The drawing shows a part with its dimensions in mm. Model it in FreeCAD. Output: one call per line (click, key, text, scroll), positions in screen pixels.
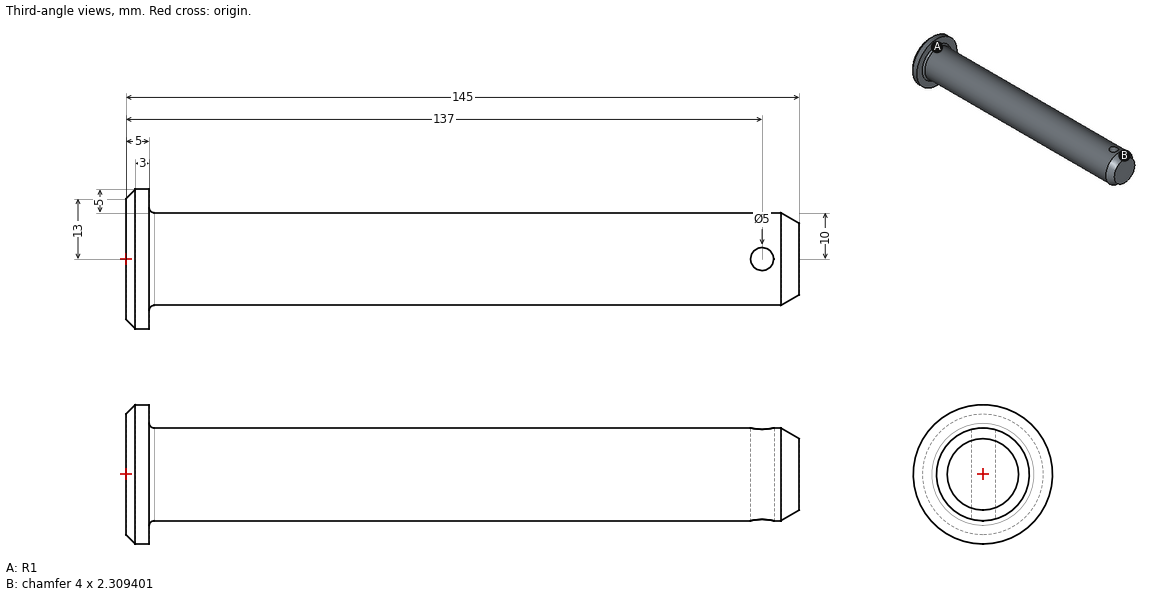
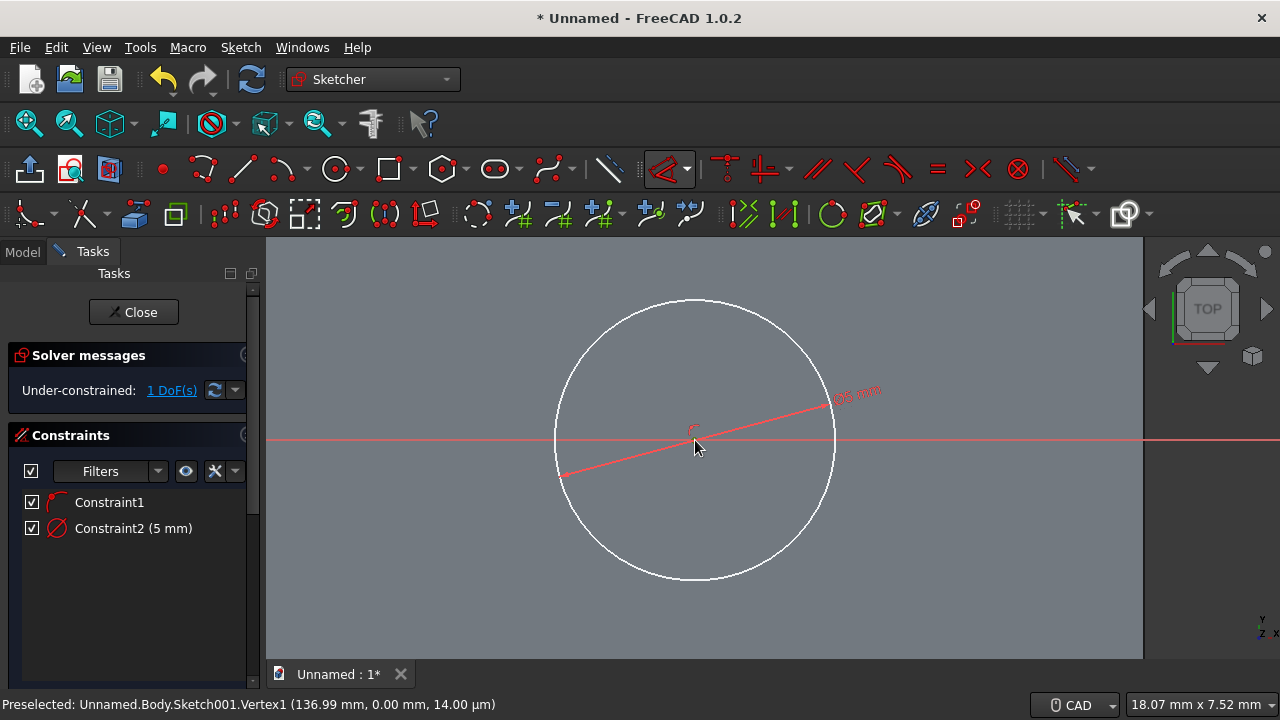
key(l)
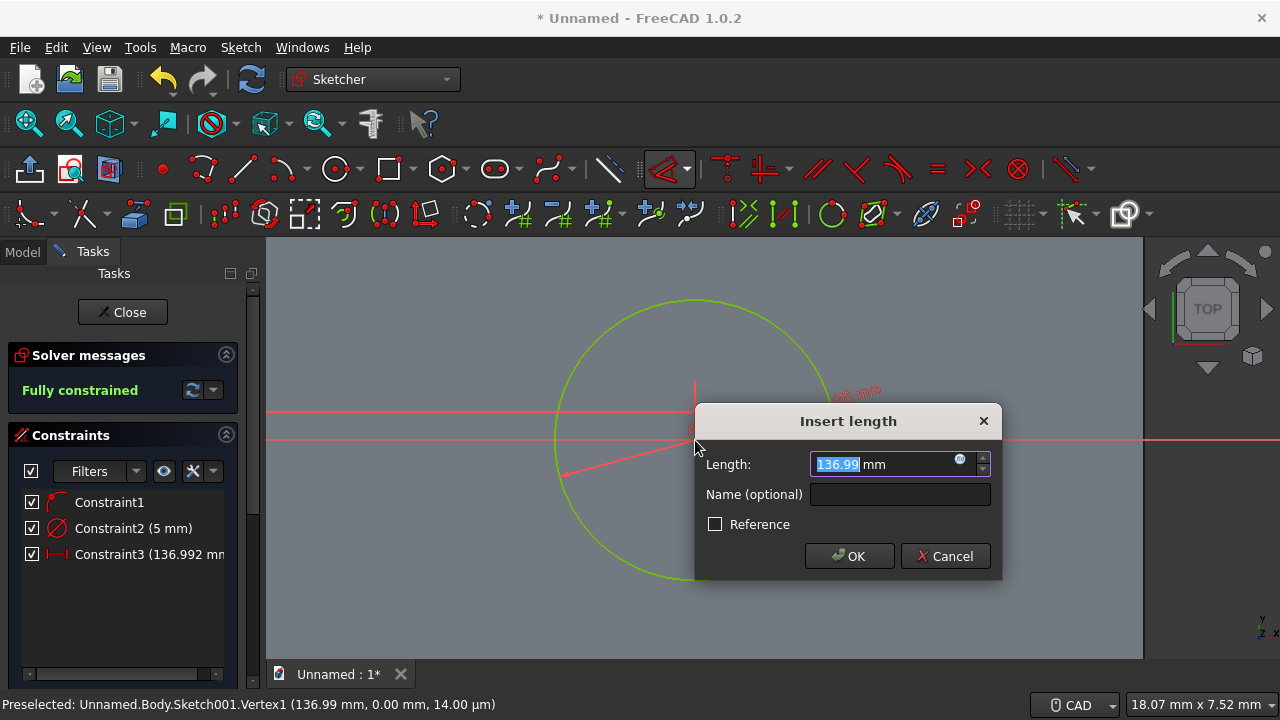
text(137)
key(Return)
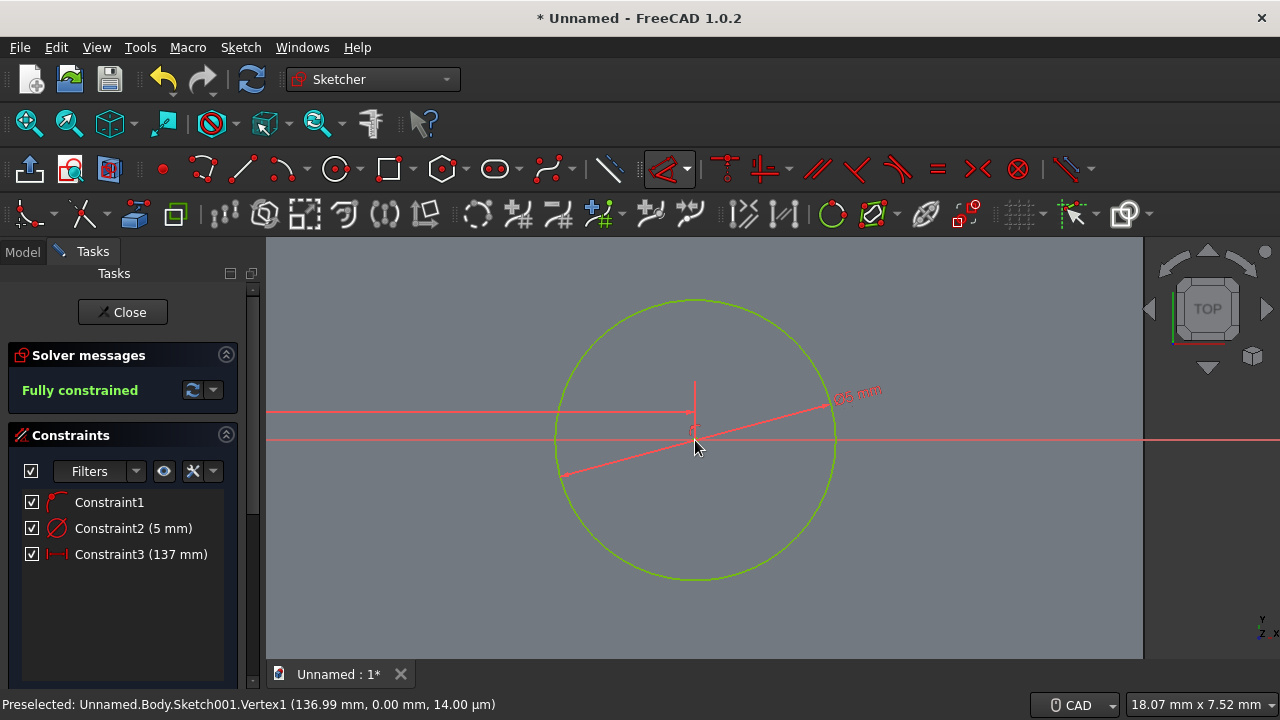
click(123, 312)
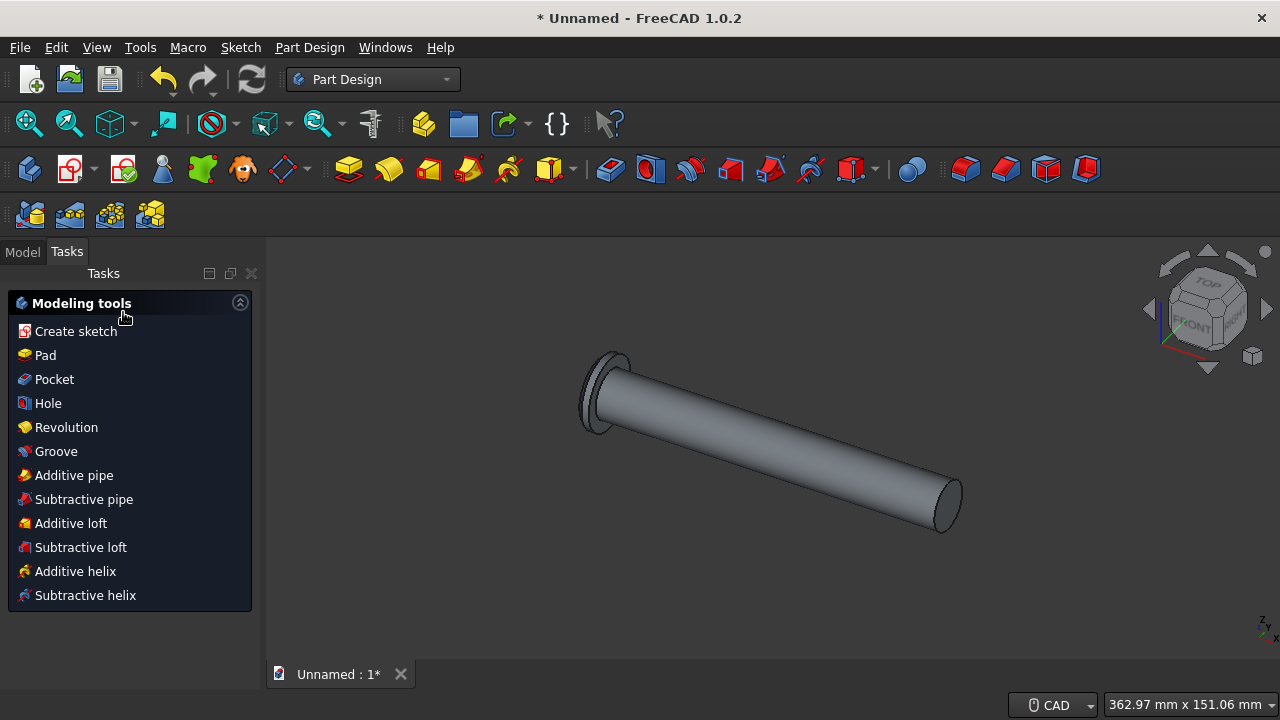
click(612, 170)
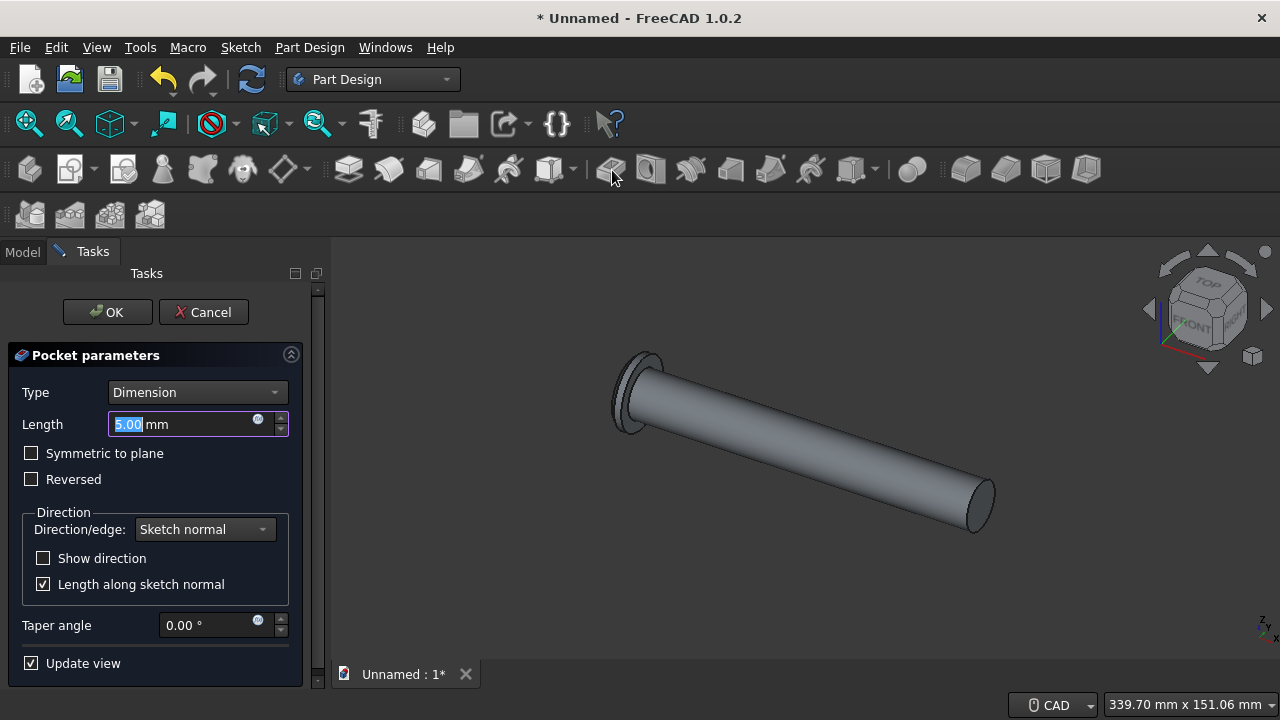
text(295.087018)
key(Tab)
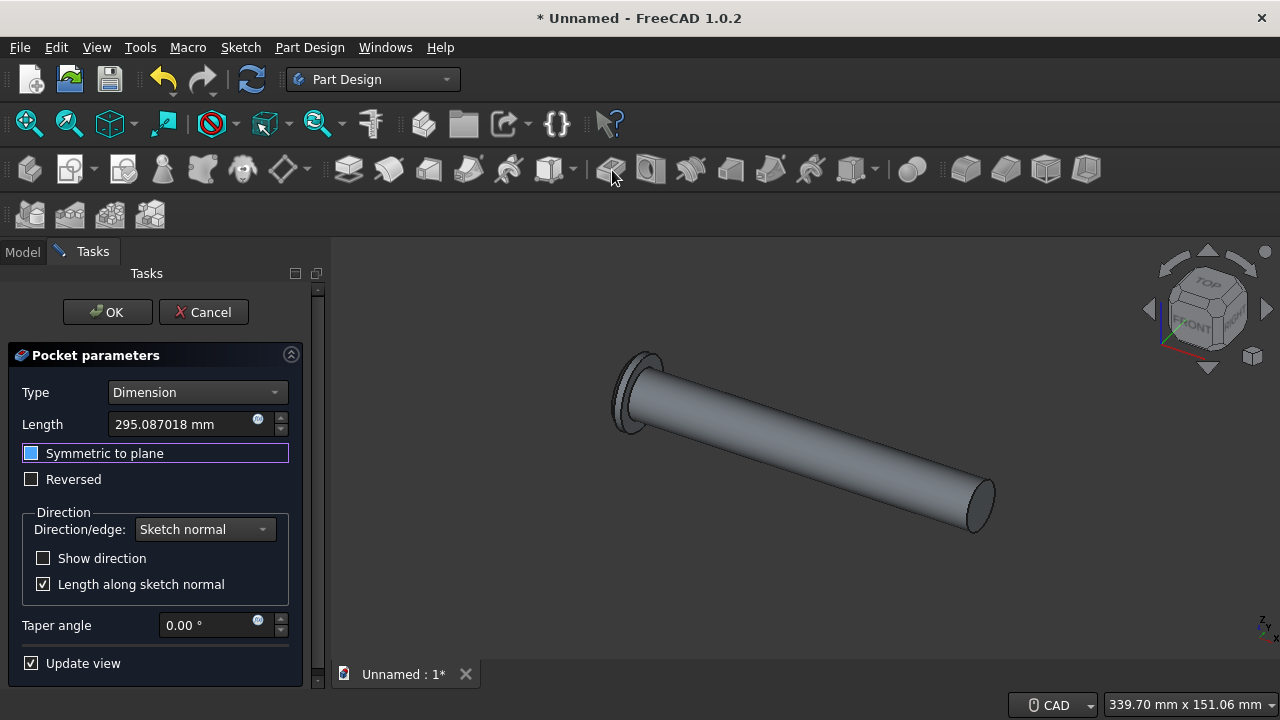
click(30, 453)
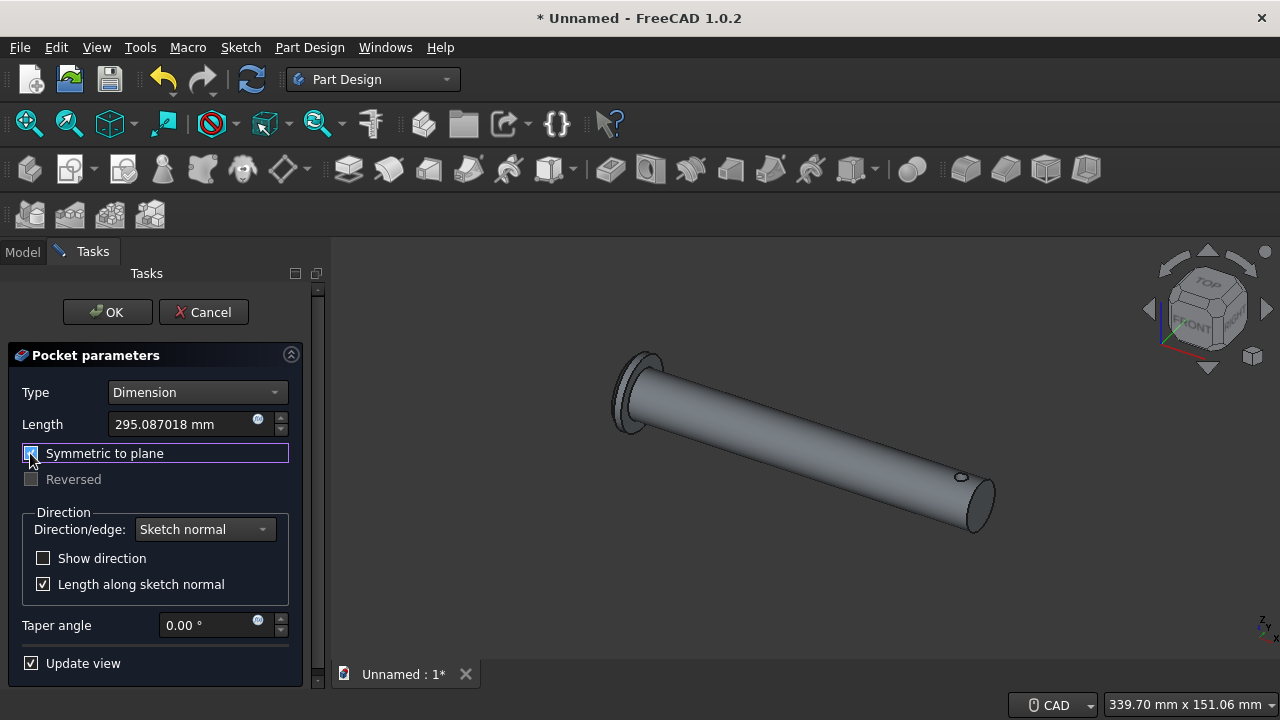
click(108, 312)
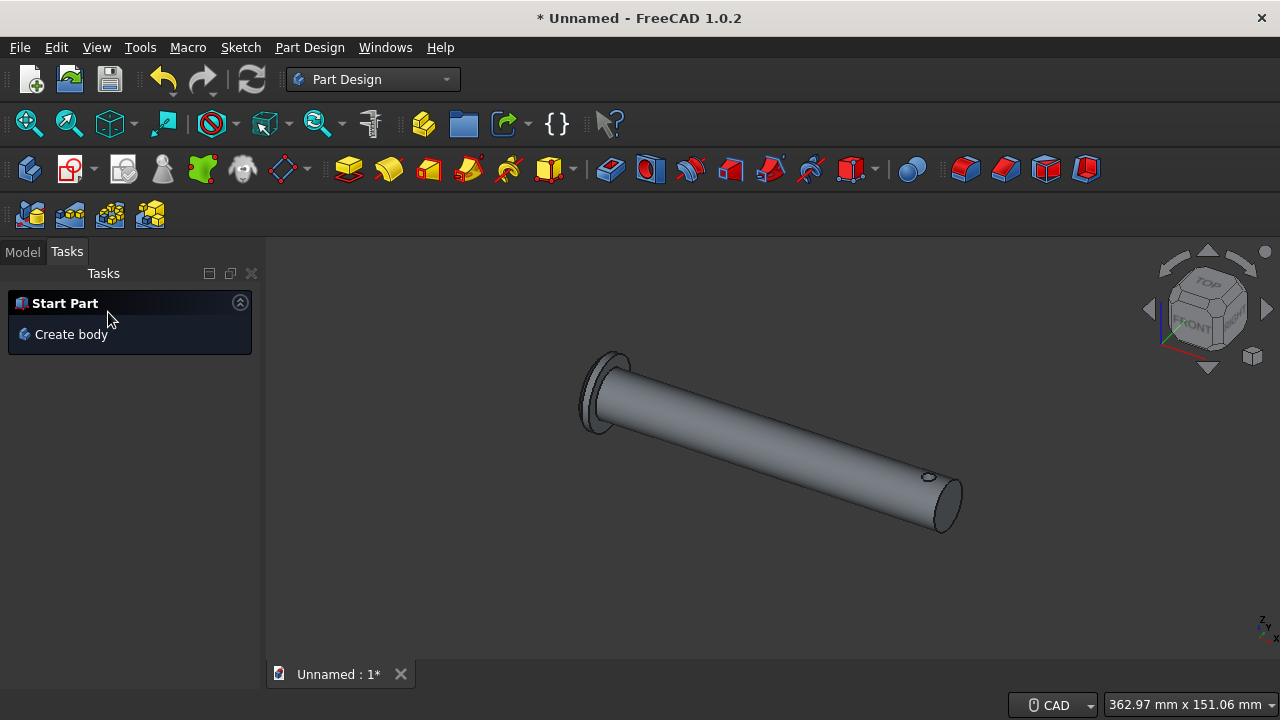
key(0)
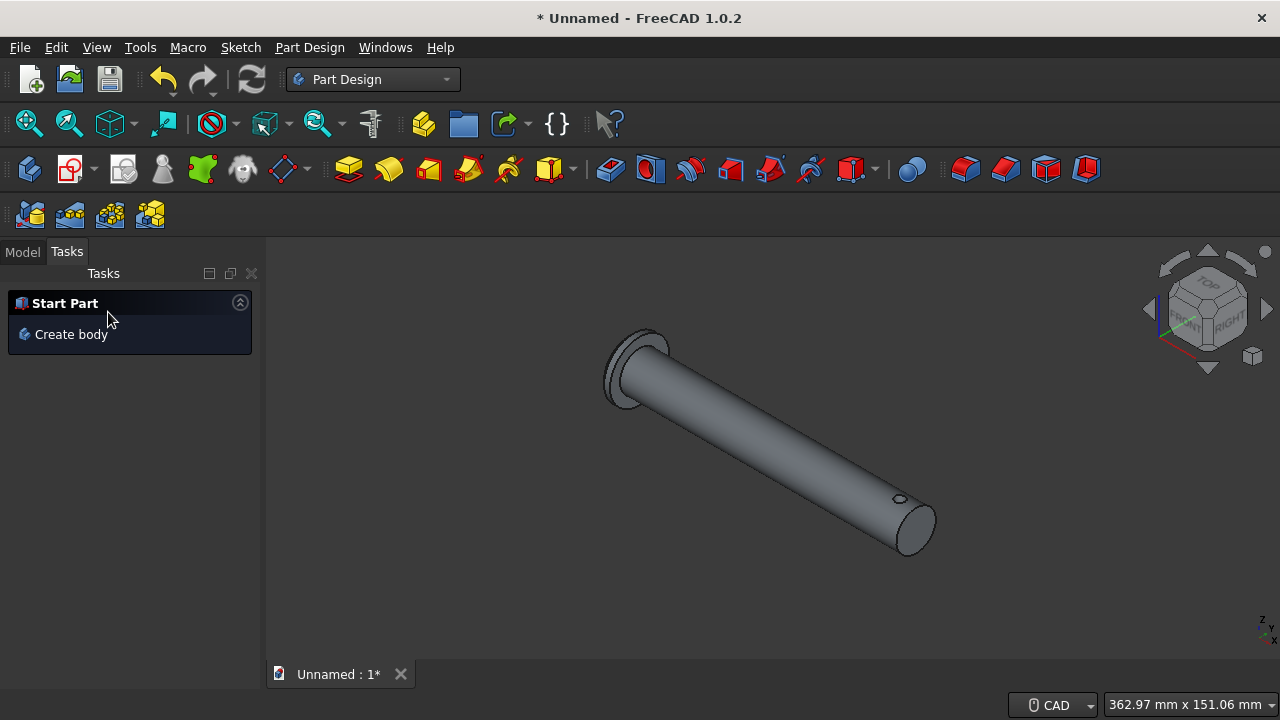
key(2)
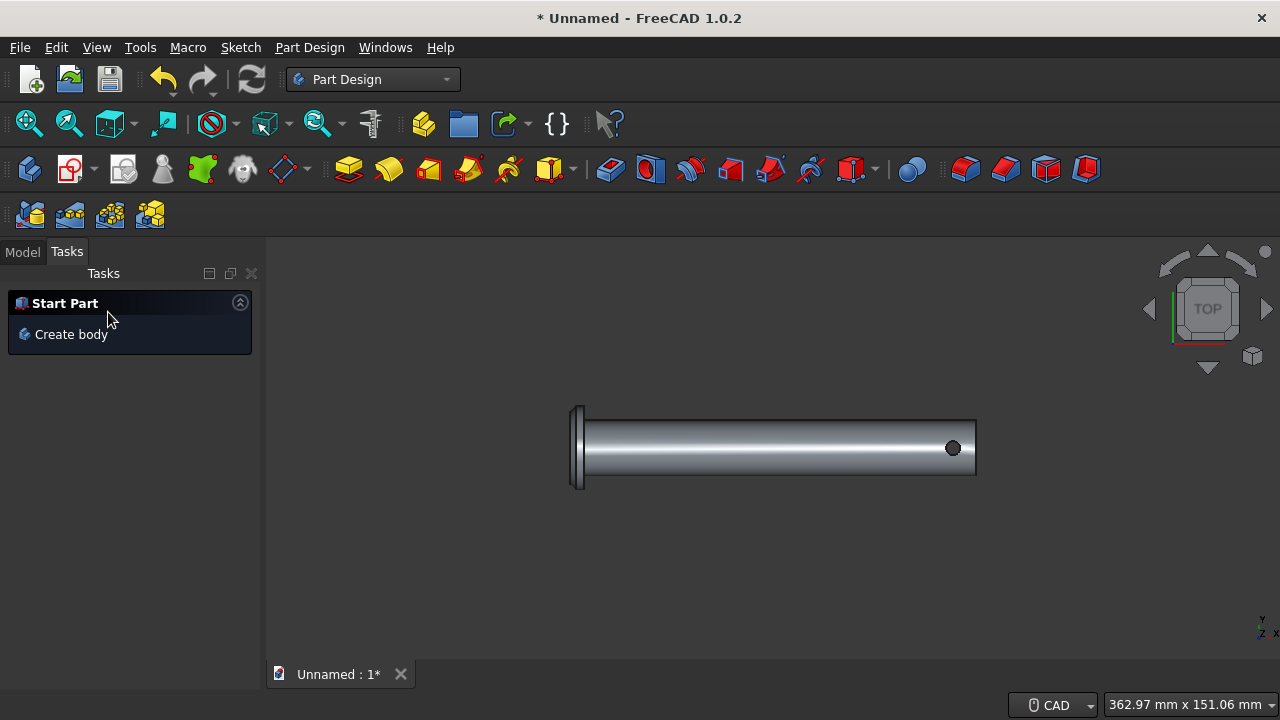
key(v)
key(f)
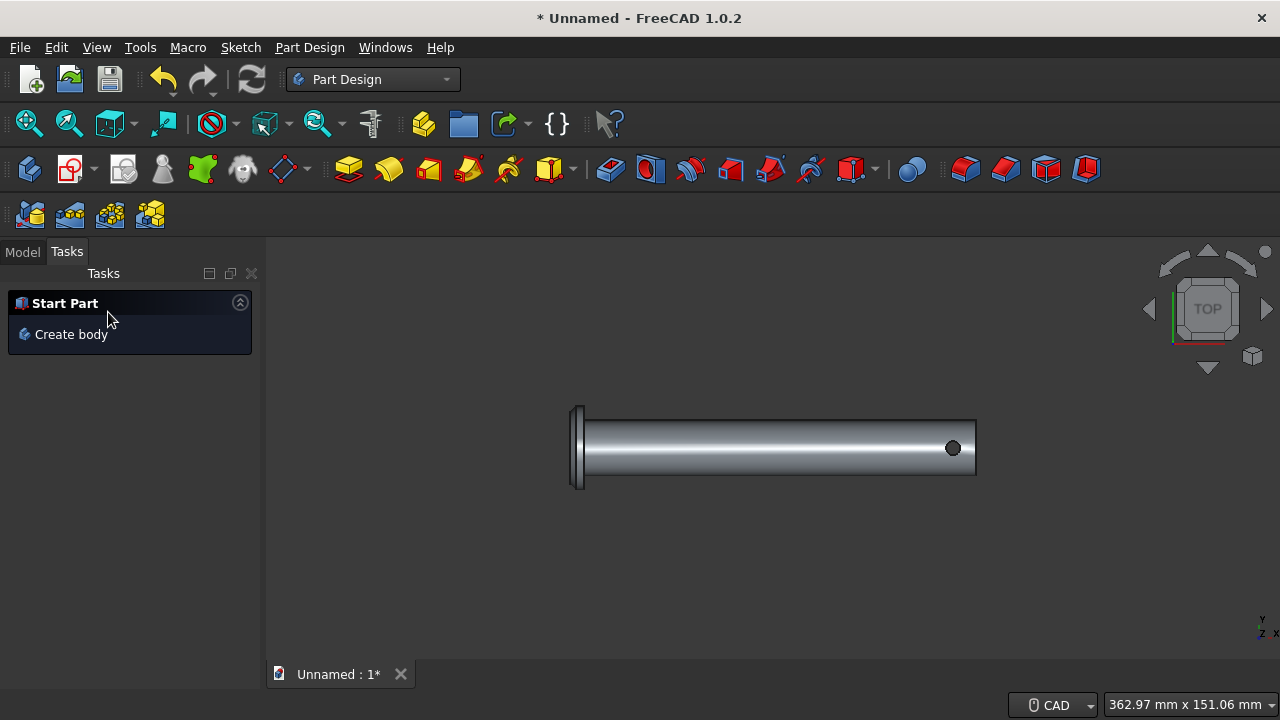
key(1)